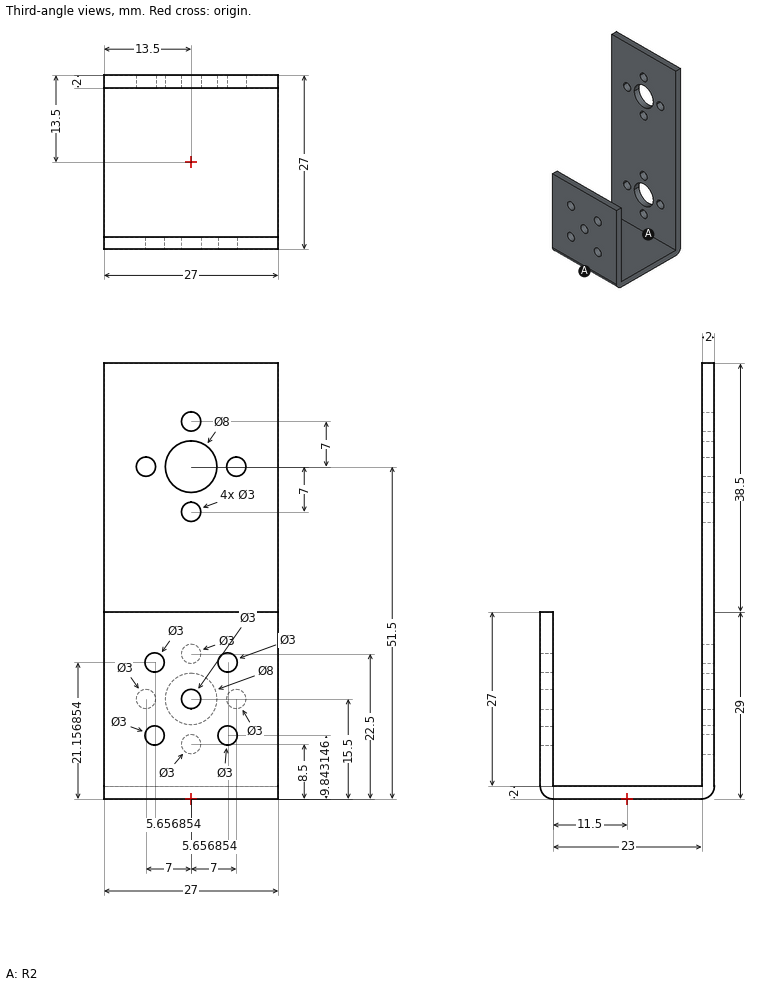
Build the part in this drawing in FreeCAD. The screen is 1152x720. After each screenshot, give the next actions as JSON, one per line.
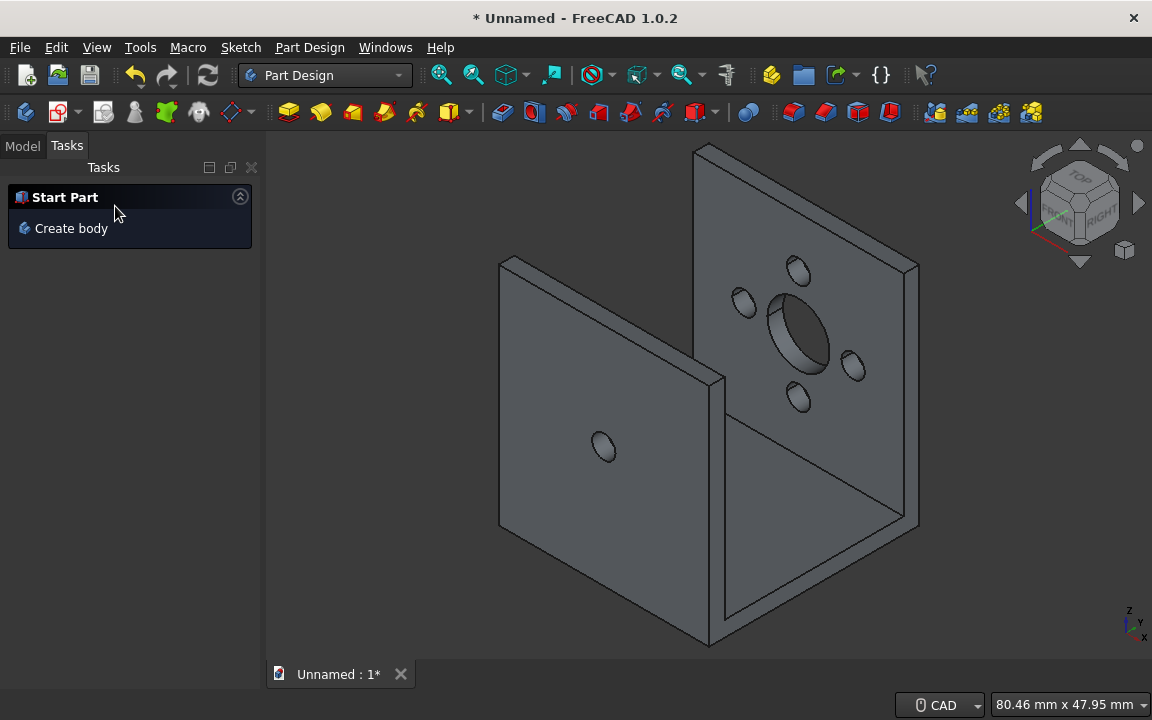
{"action": "left_click", "coordinate": [634, 398]}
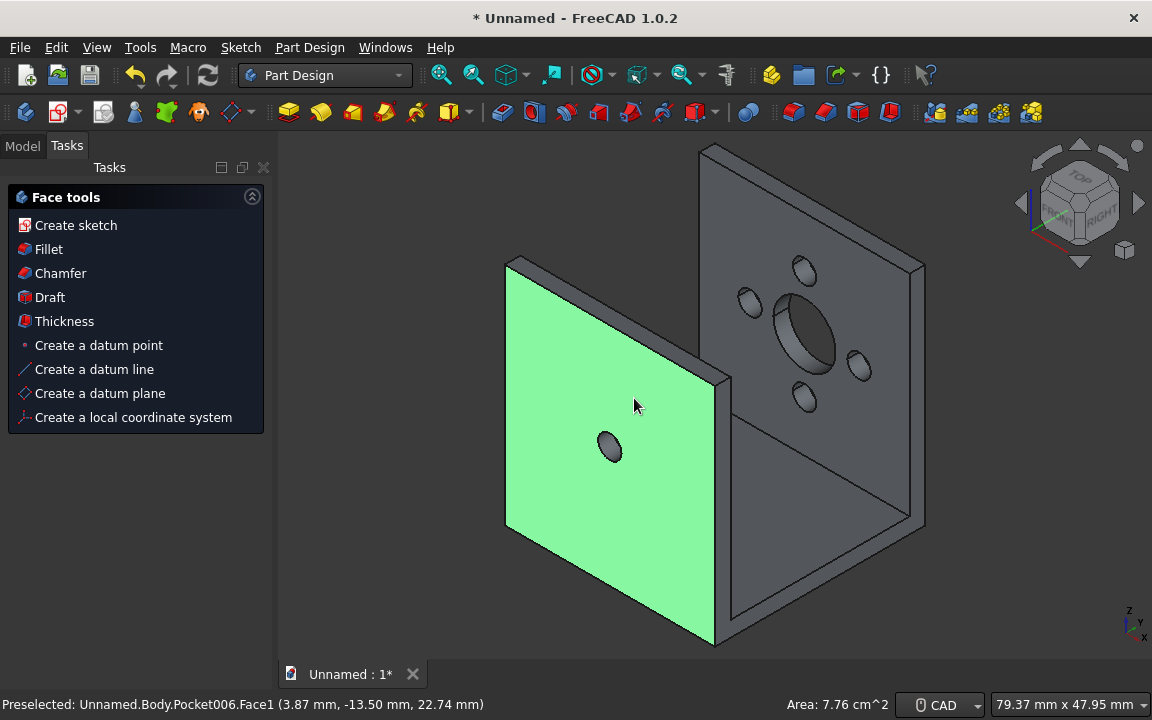
{"action": "left_click", "coordinate": [58, 112]}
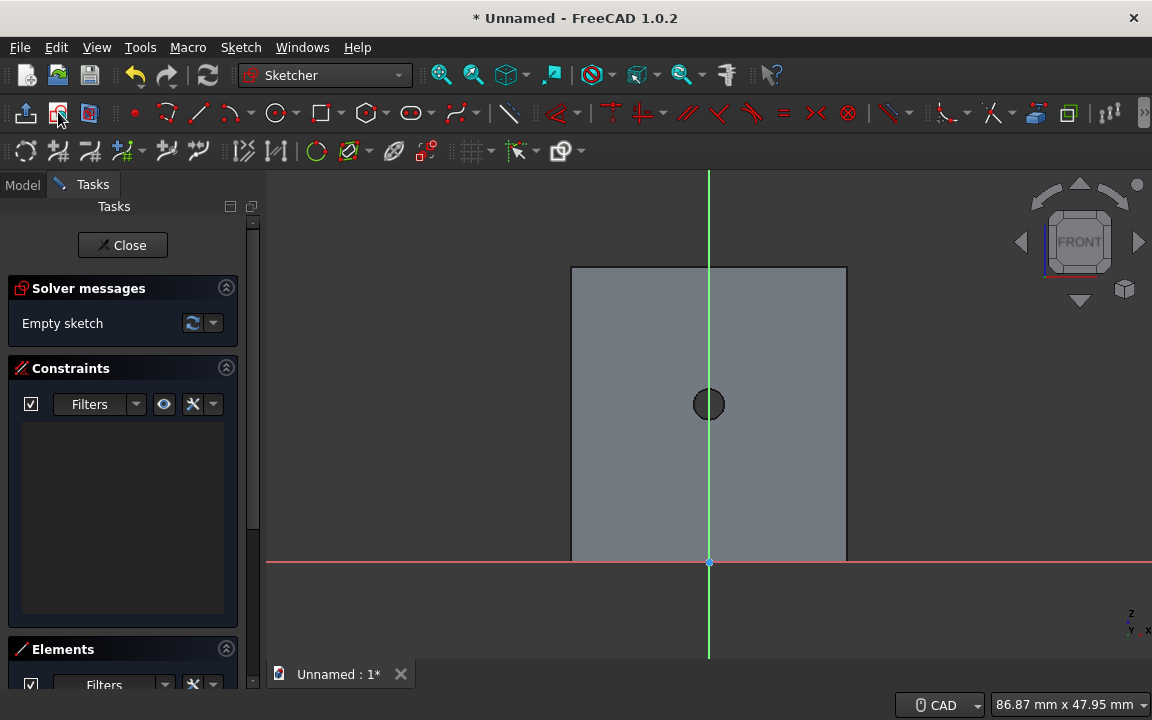
{"action": "scroll", "coordinate": [652, 340], "scroll_direction": "up", "scroll_amount": 12}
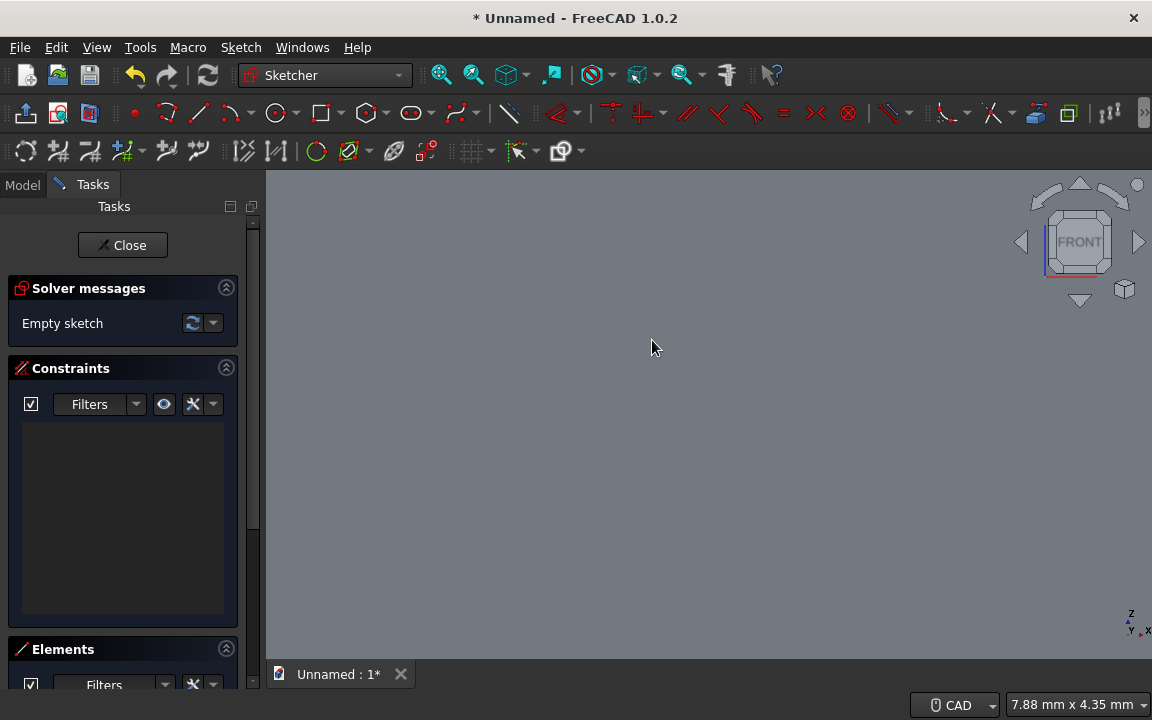
{"action": "key", "text": "g c"}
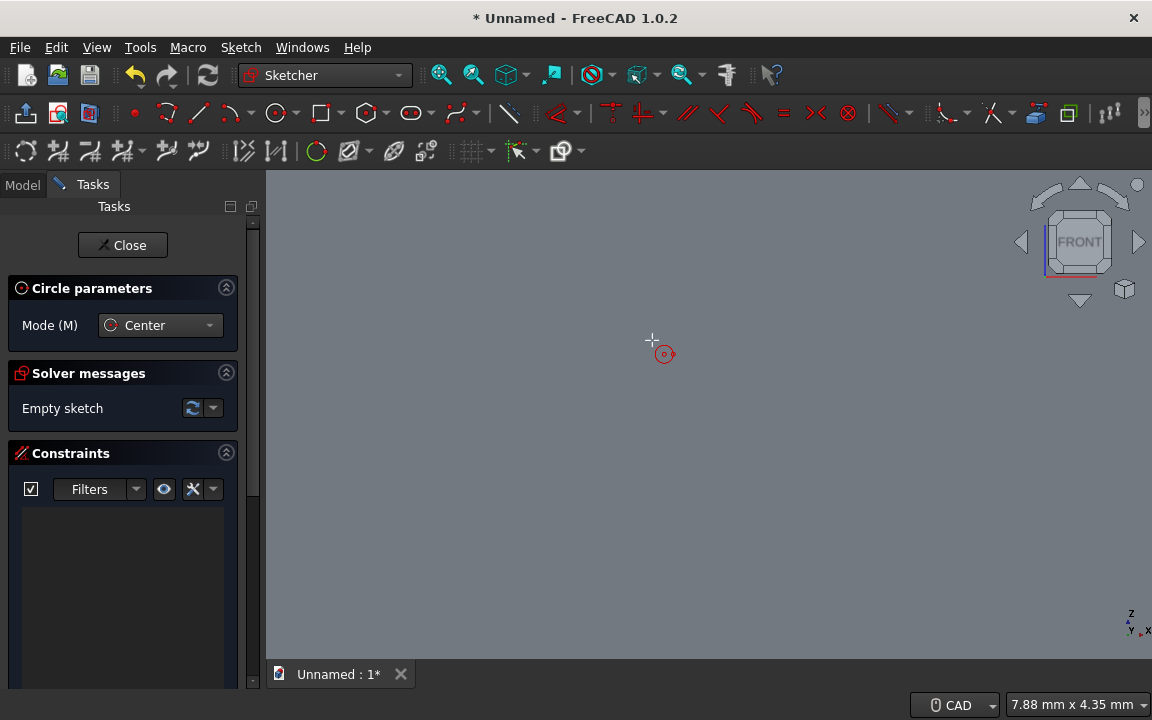
{"action": "left_click", "coordinate": [640, 409]}
{"action": "left_click", "coordinate": [759, 290]}
{"action": "key", "text": "Escape"}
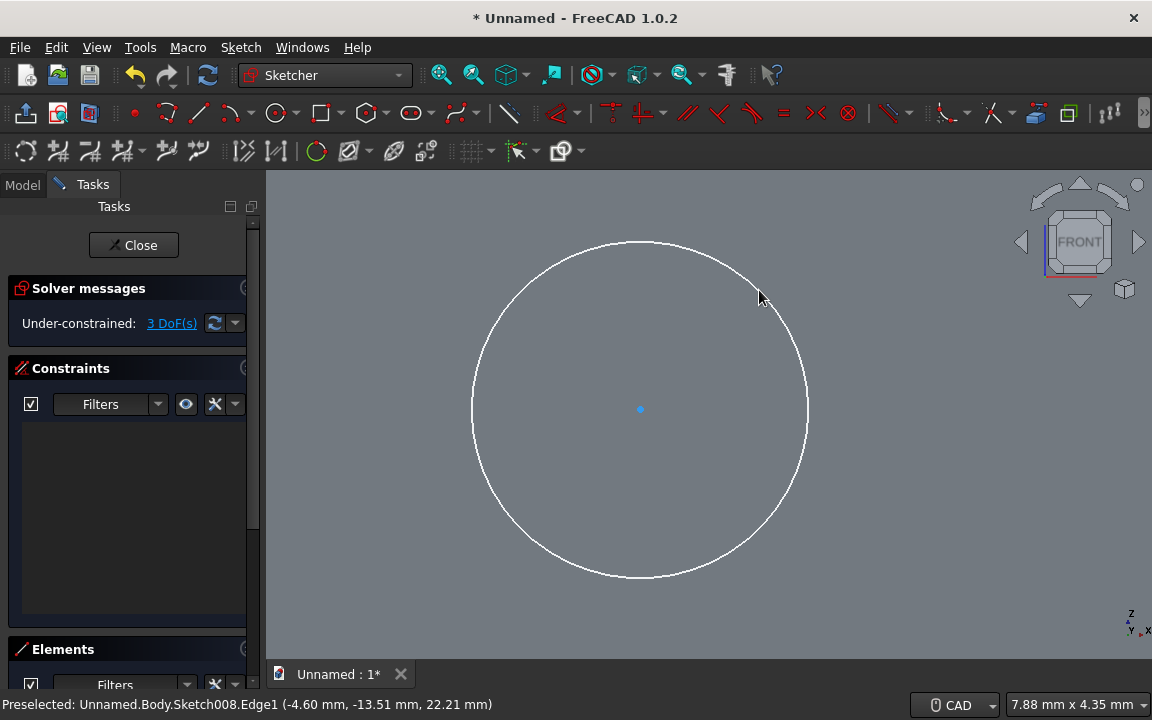
{"action": "left_click", "coordinate": [556, 114]}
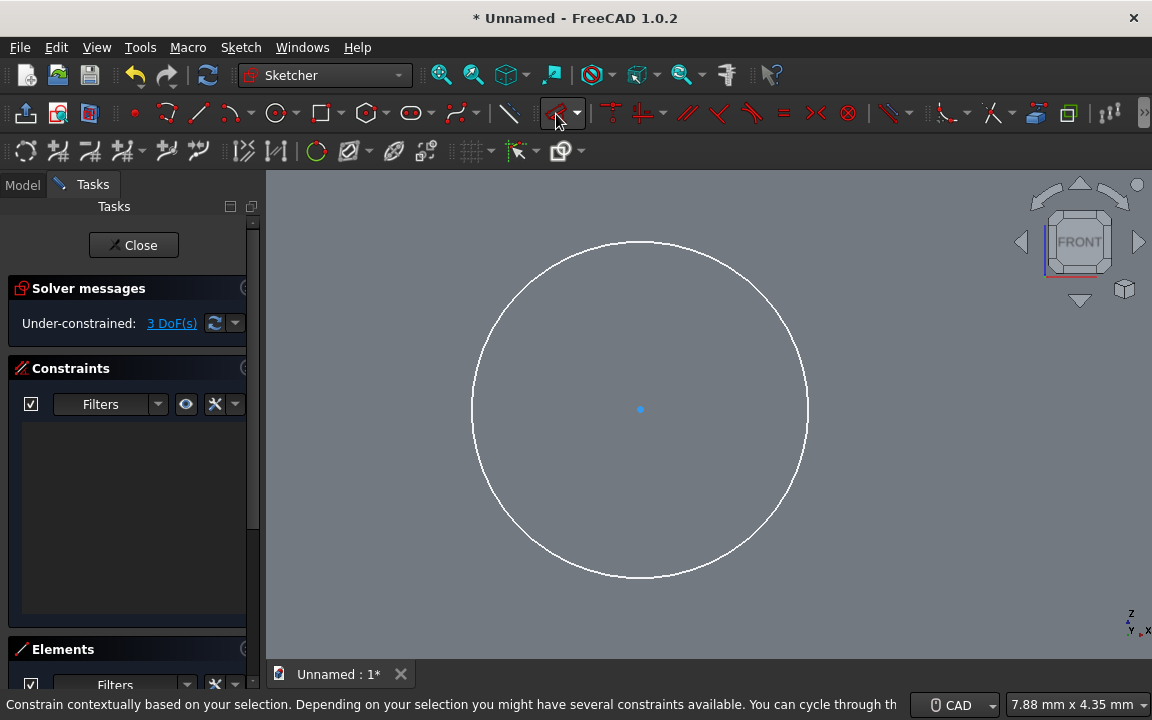
{"action": "left_click", "coordinate": [759, 291]}
{"action": "left_click", "coordinate": [782, 268]}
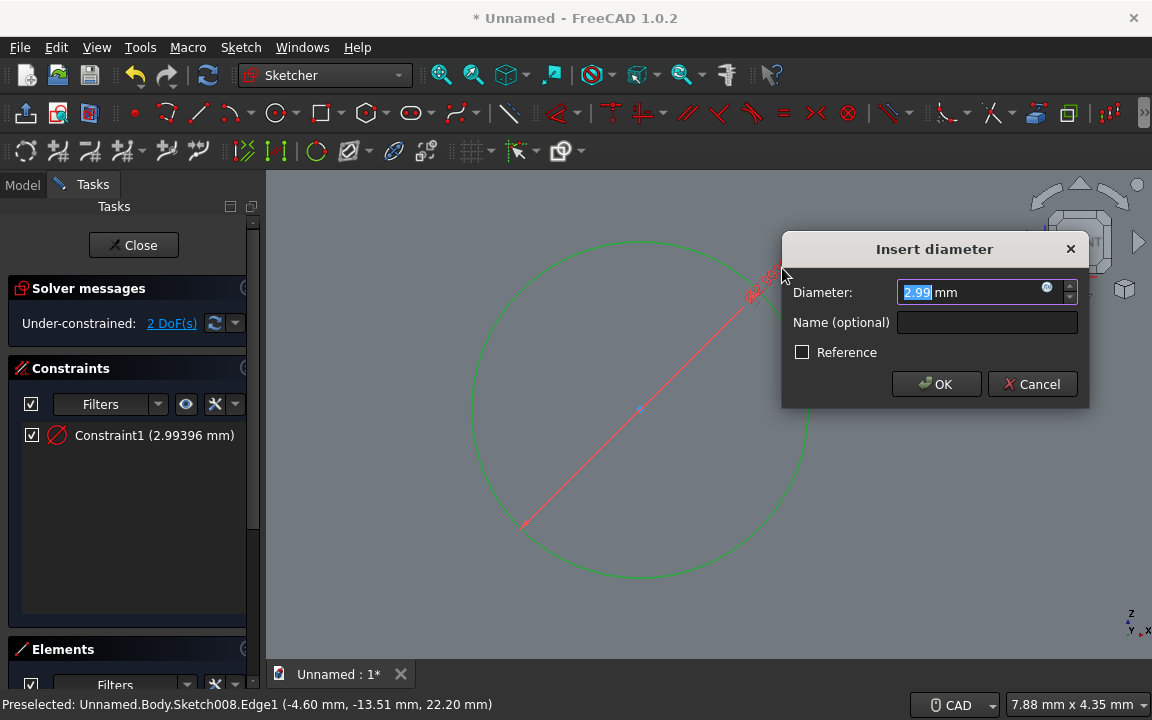
{"action": "type", "text": "3"}
{"action": "key", "text": "Return"}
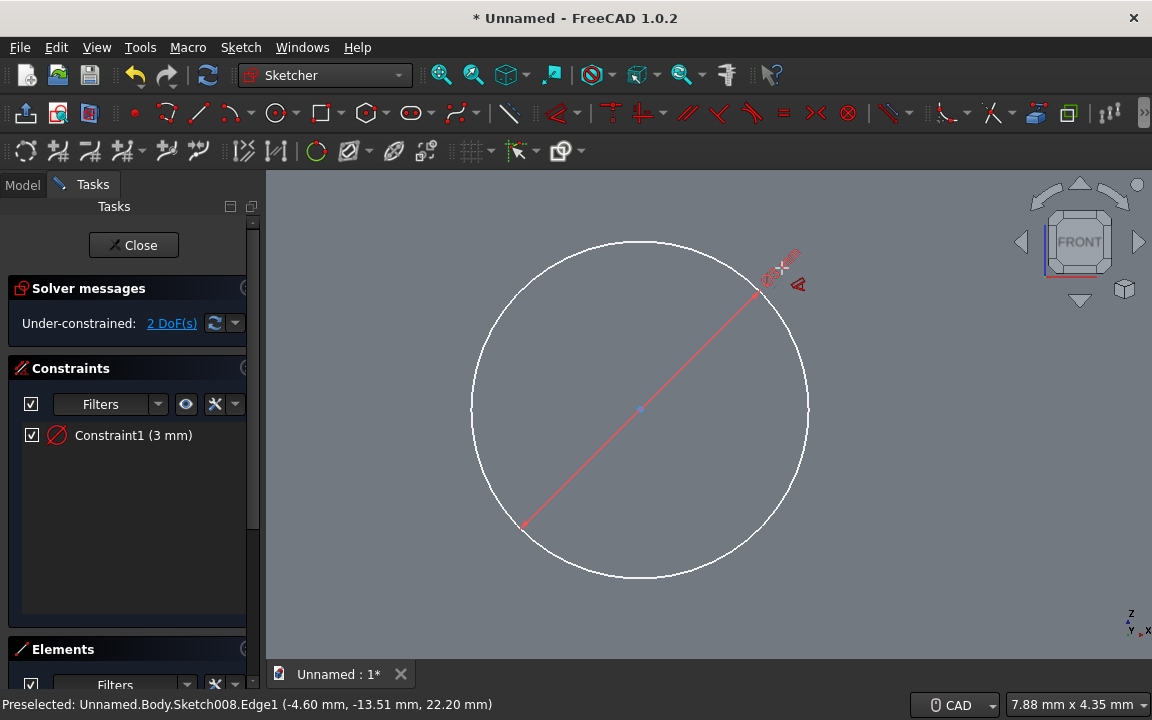
{"action": "left_click", "coordinate": [640, 410]}
{"action": "left_click", "coordinate": [734, 376]}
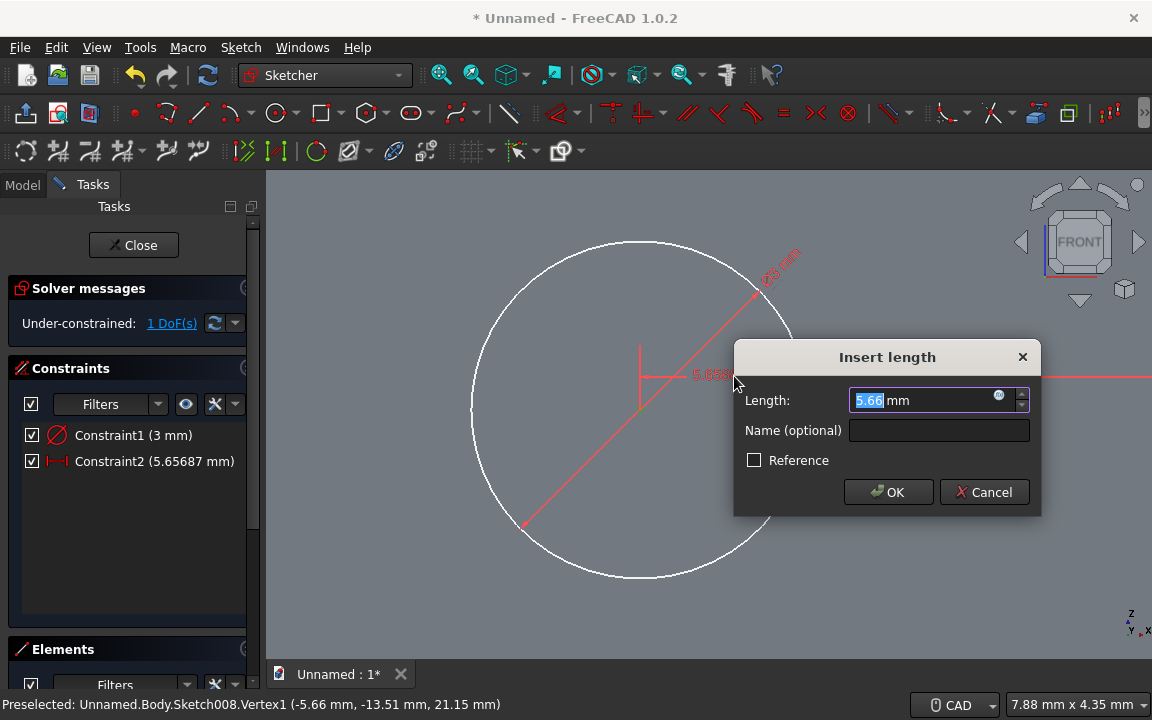
{"action": "type", "text": "5.656854"}
{"action": "key", "text": "Return"}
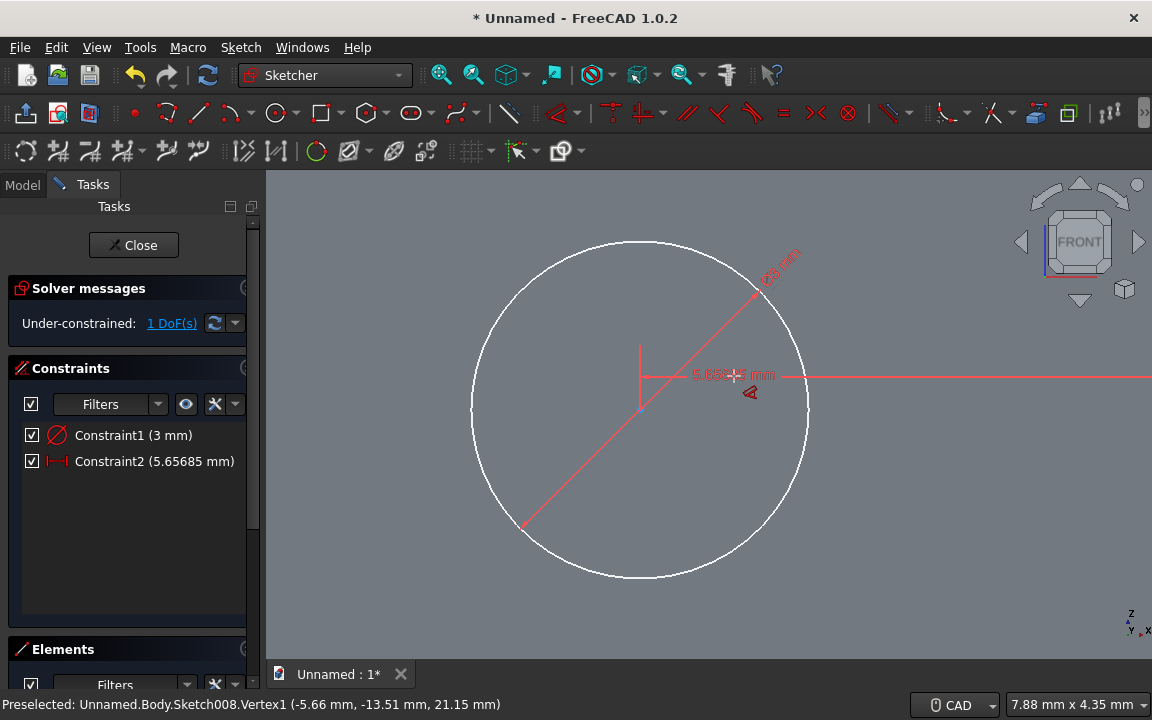
{"action": "left_click", "coordinate": [640, 410]}
{"action": "left_click", "coordinate": [606, 521]}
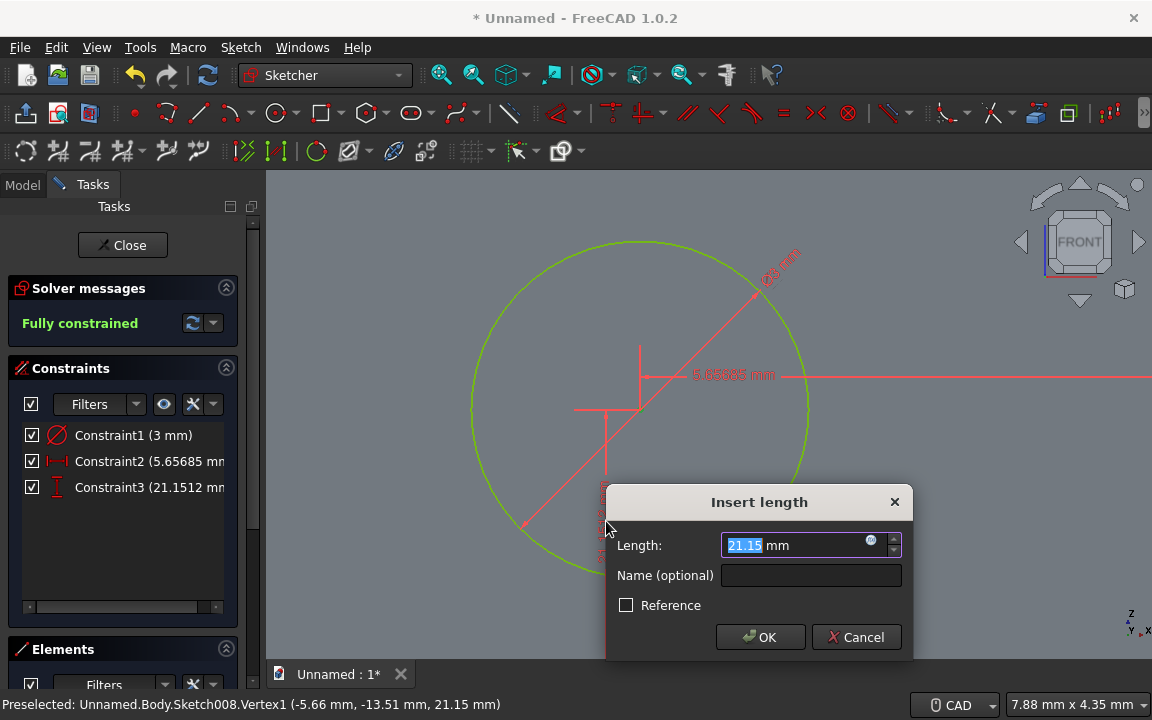
{"action": "type", "text": "21.156854"}
{"action": "key", "text": "Return"}
{"action": "key", "text": "Escape"}